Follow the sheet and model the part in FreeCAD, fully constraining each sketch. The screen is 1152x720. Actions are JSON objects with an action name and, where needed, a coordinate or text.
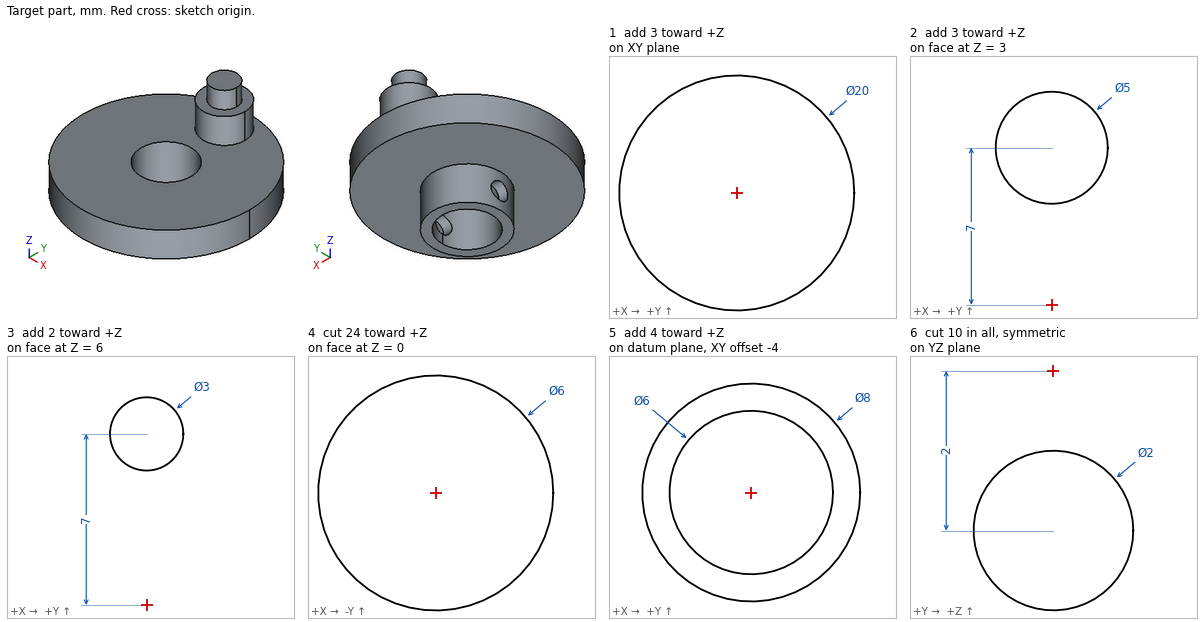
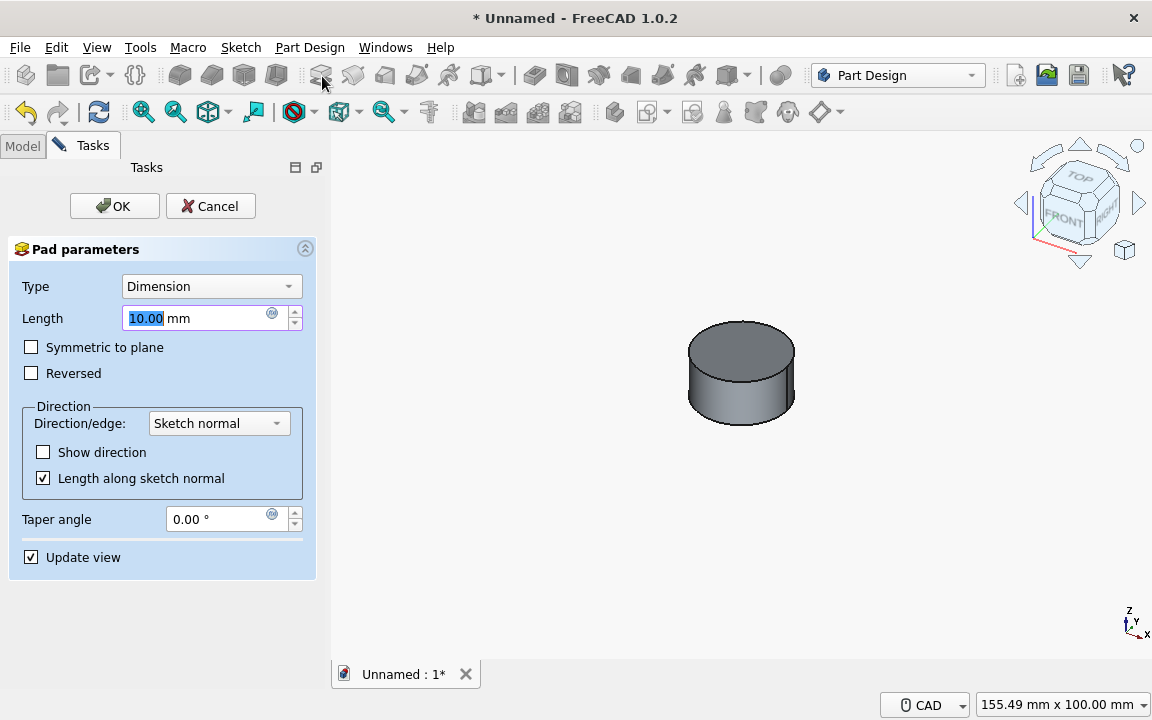
{"action": "type", "text": "3"}
{"action": "key", "text": "Tab"}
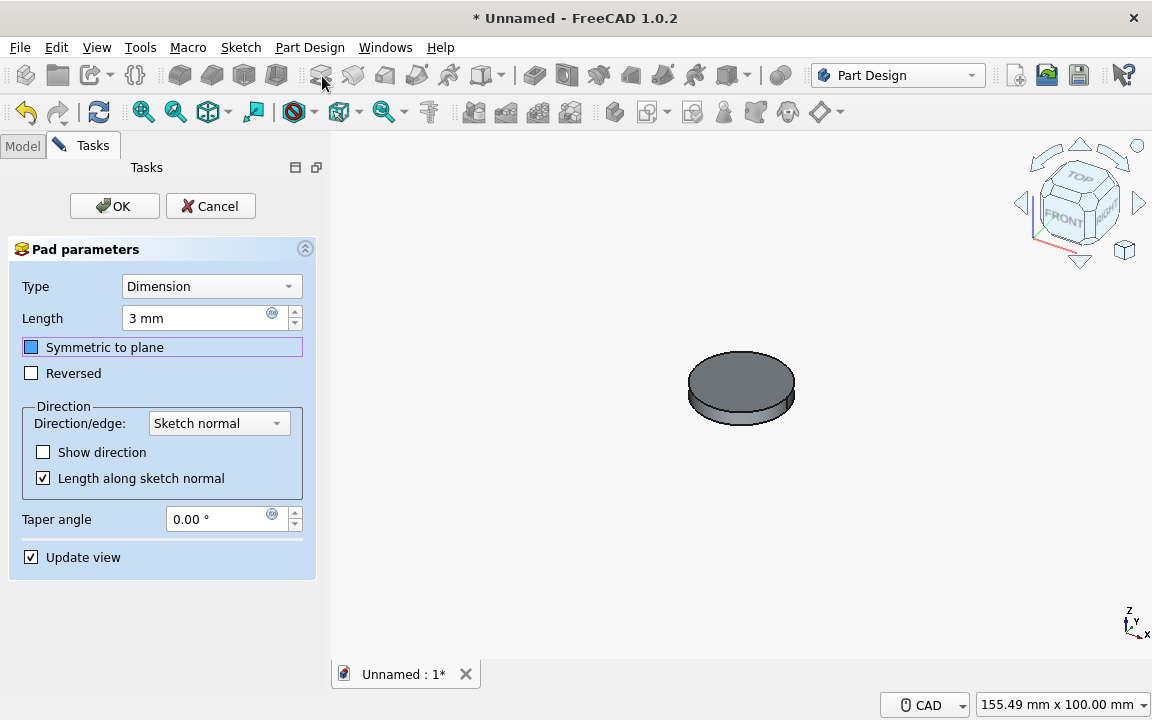
{"action": "left_click", "coordinate": [115, 206]}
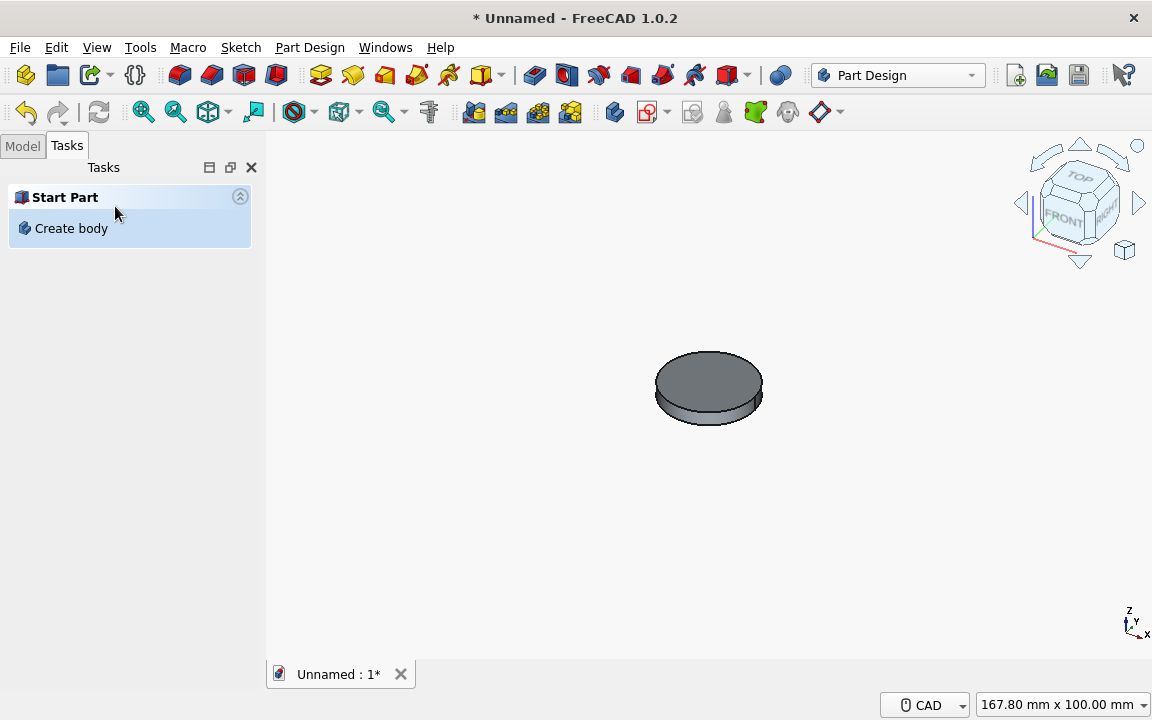
{"action": "key", "text": "v f"}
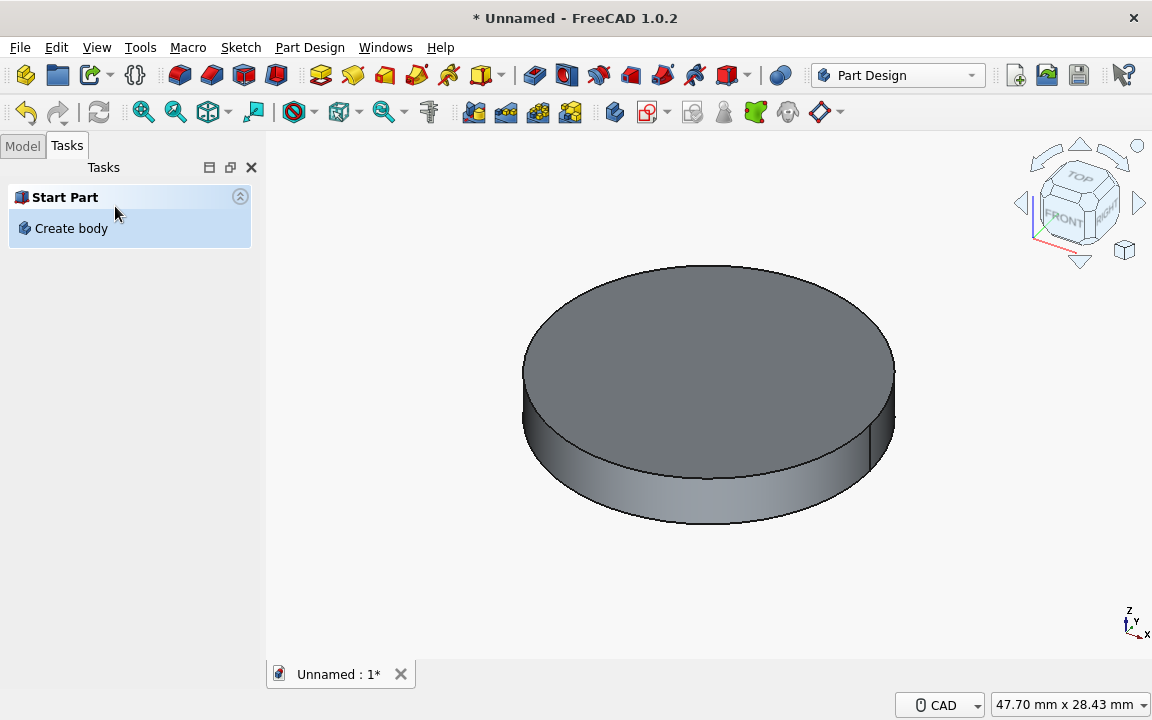
{"action": "left_click", "coordinate": [709, 371]}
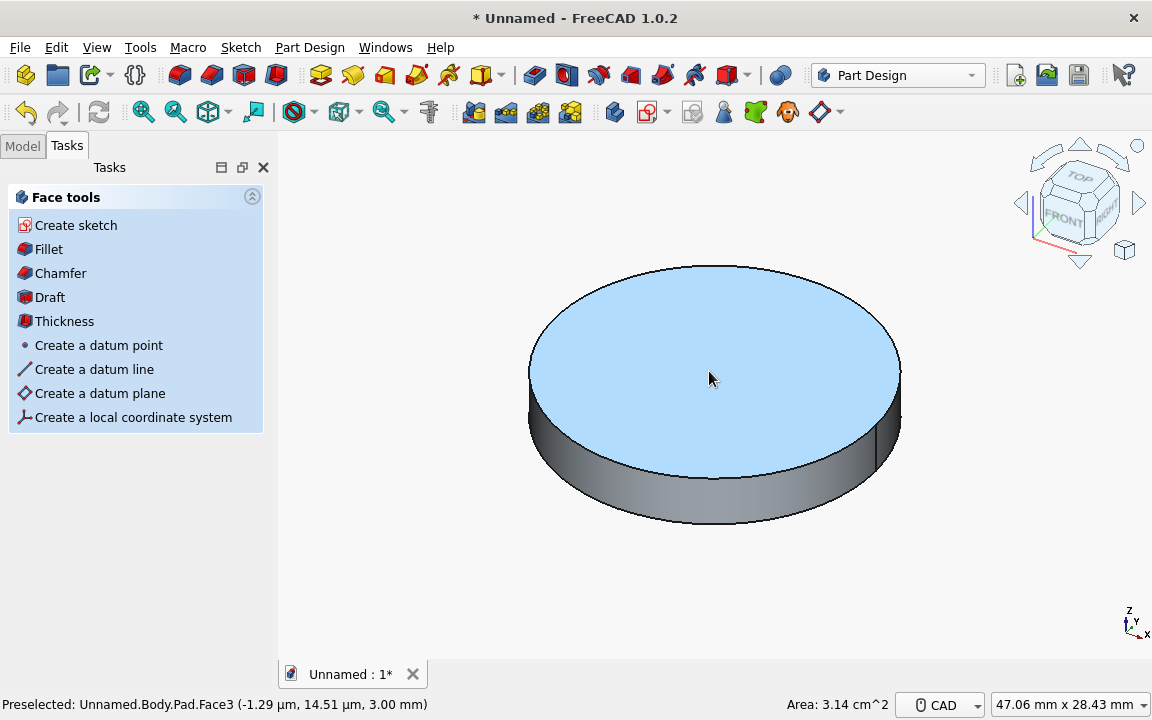
{"action": "left_click", "coordinate": [648, 112]}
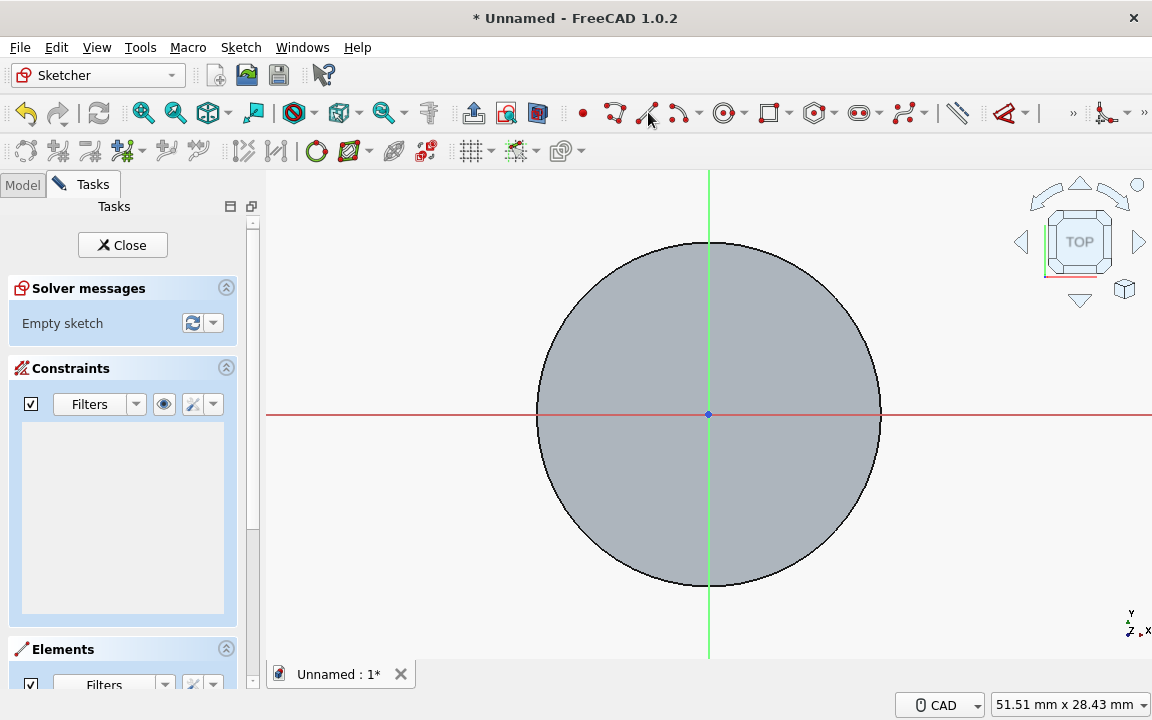
{"action": "scroll", "coordinate": [792, 233], "scroll_direction": "up", "scroll_amount": 3}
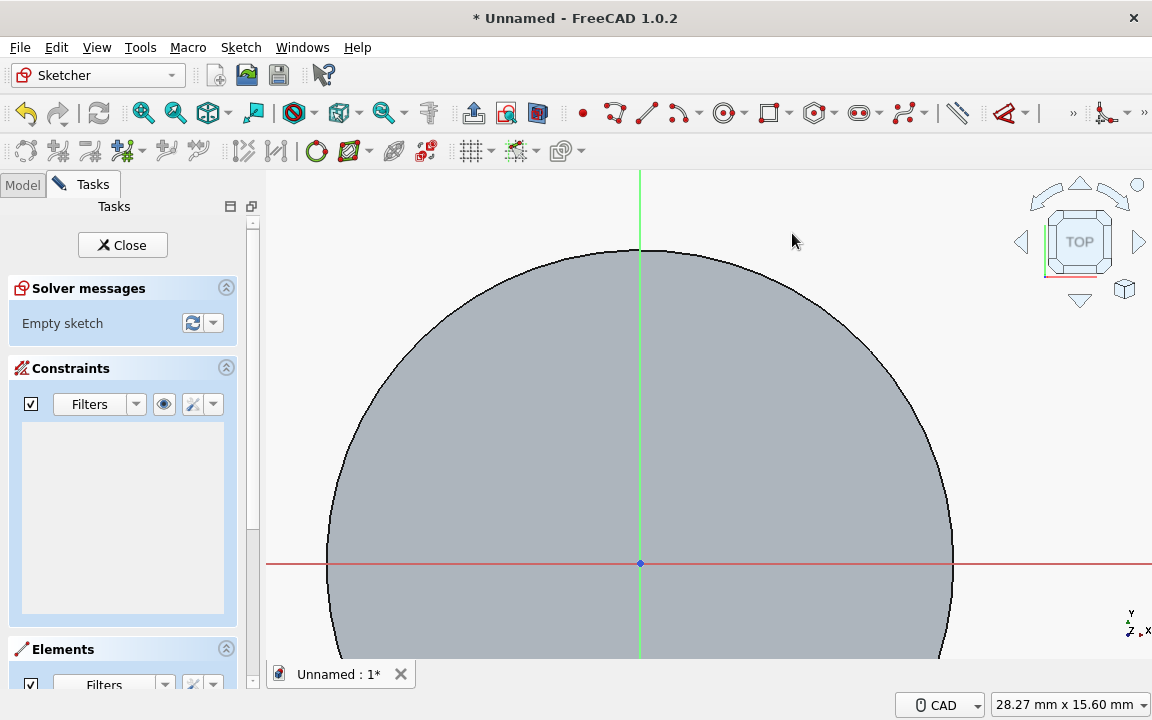
{"action": "left_click", "coordinate": [724, 114]}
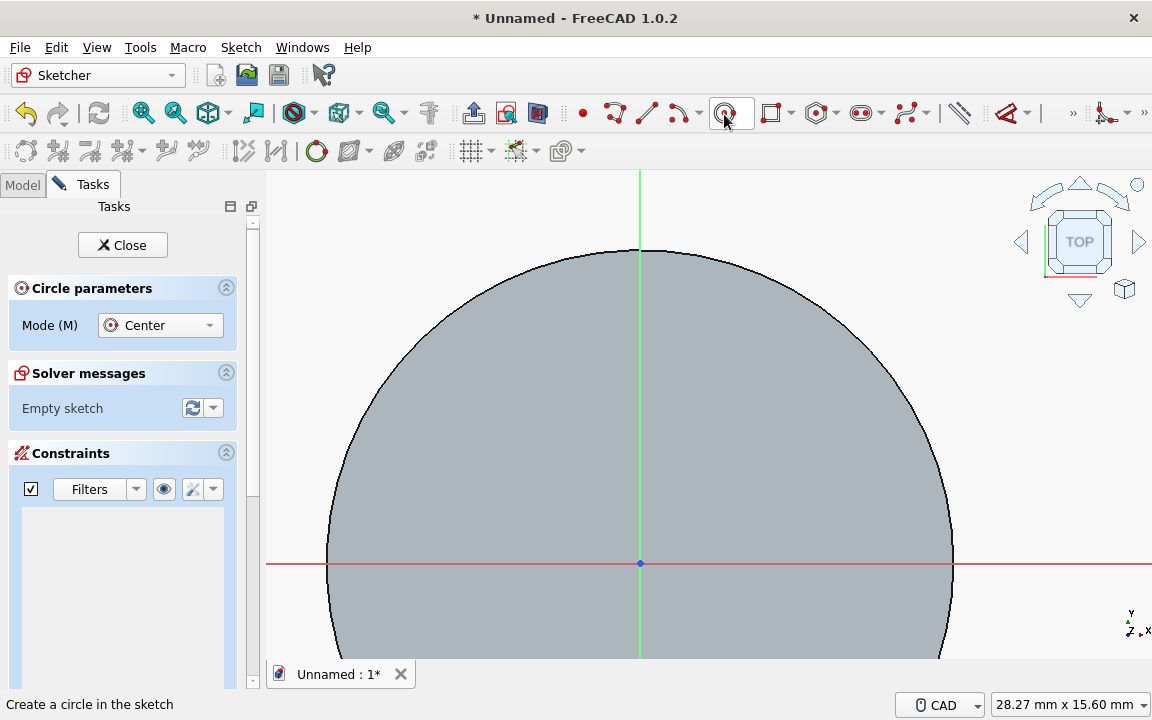
{"action": "left_click", "coordinate": [640, 344]}
{"action": "left_click", "coordinate": [695, 289]}
{"action": "key", "text": "Escape"}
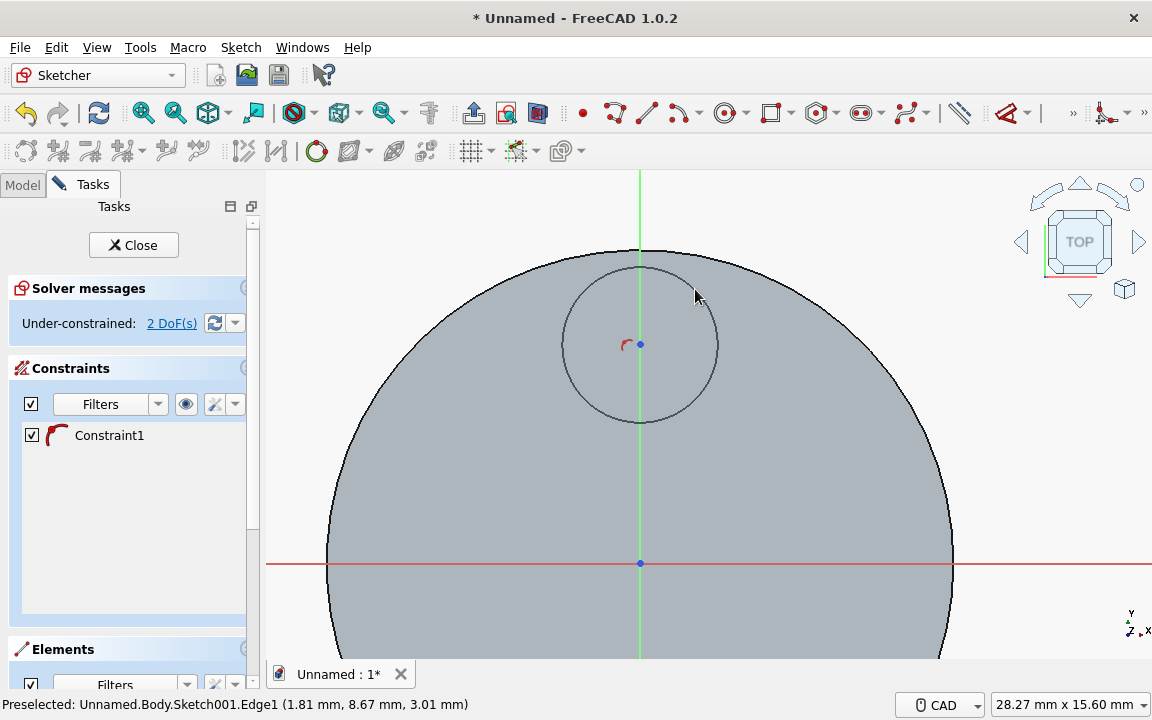
{"action": "left_click", "coordinate": [1006, 114]}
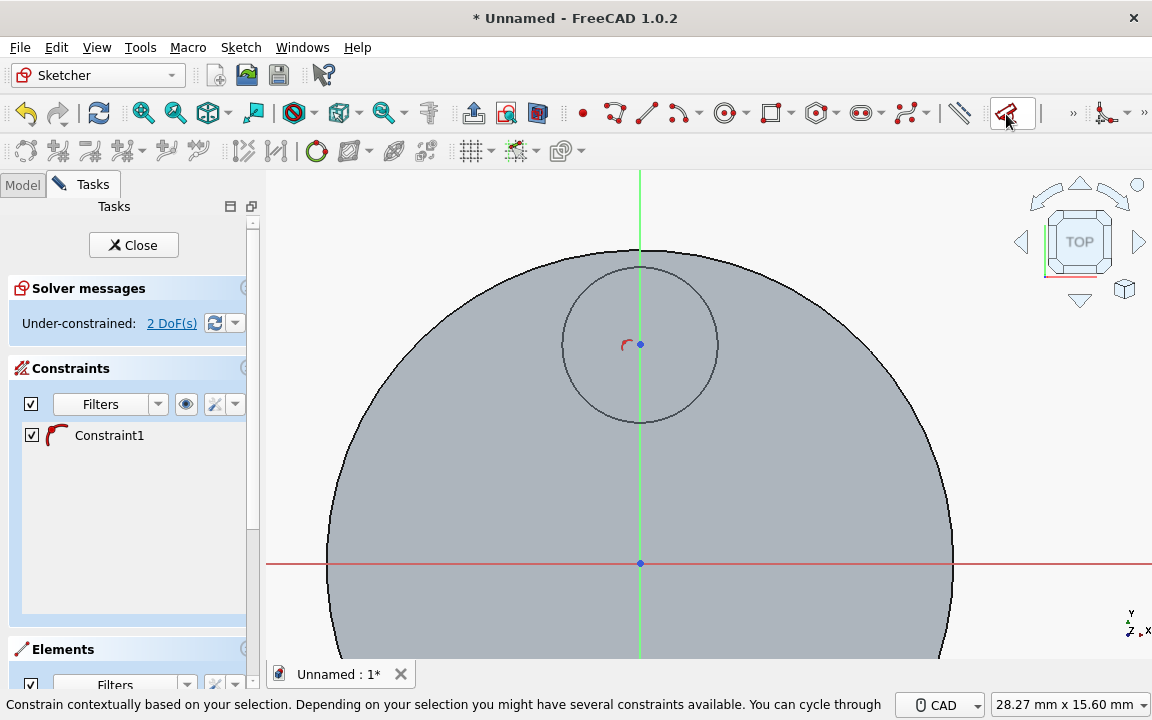
{"action": "left_click", "coordinate": [695, 290]}
{"action": "left_click", "coordinate": [718, 267]}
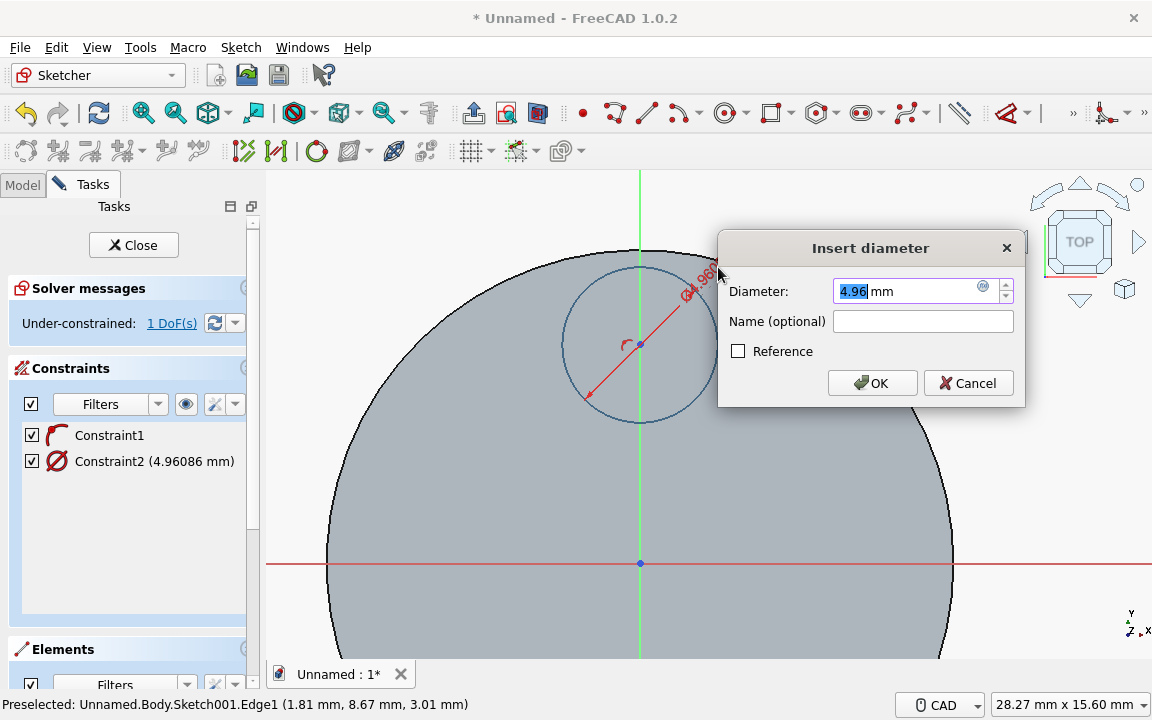
{"action": "type", "text": "5"}
{"action": "key", "text": "Return"}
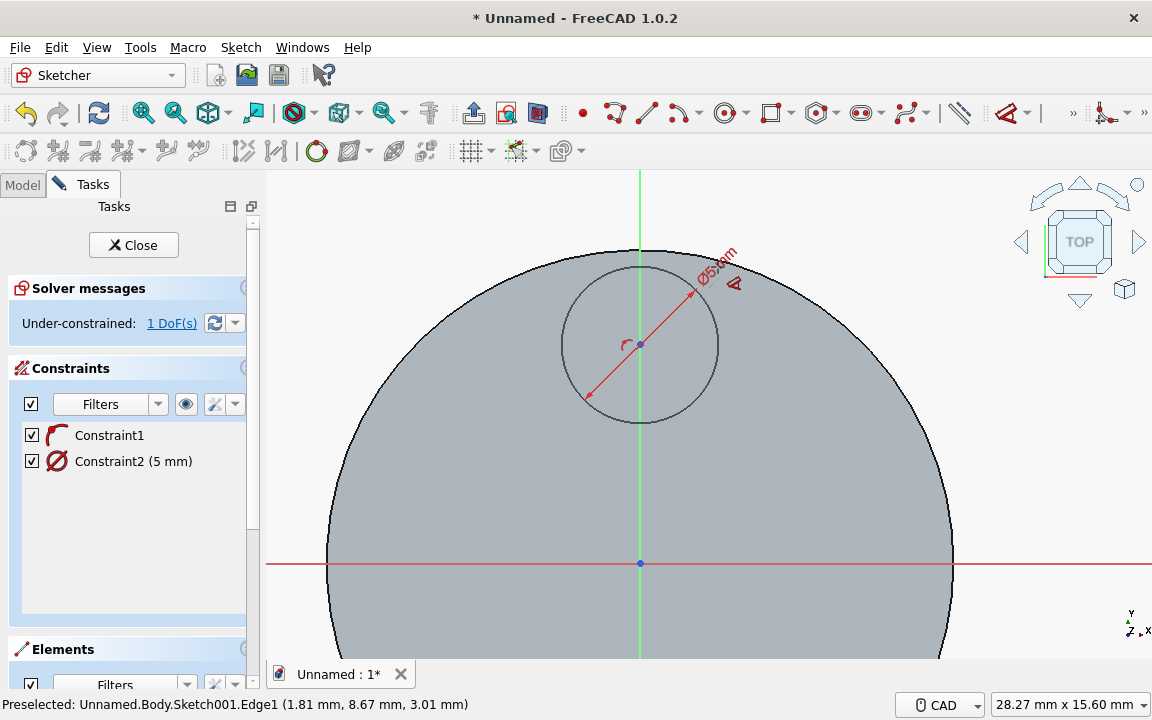
{"action": "left_click", "coordinate": [640, 345]}
{"action": "left_click", "coordinate": [674, 454]}